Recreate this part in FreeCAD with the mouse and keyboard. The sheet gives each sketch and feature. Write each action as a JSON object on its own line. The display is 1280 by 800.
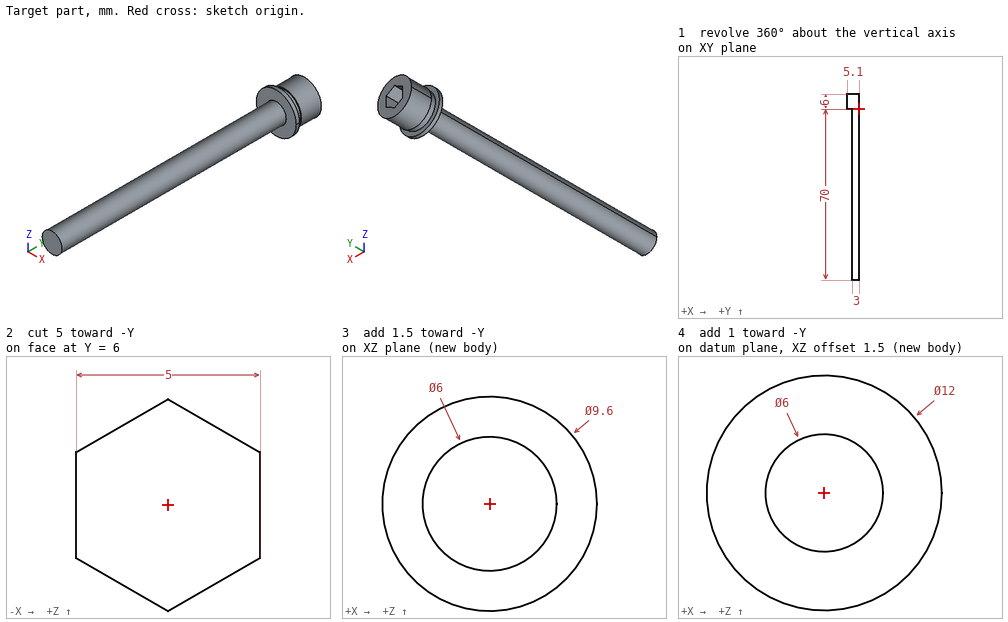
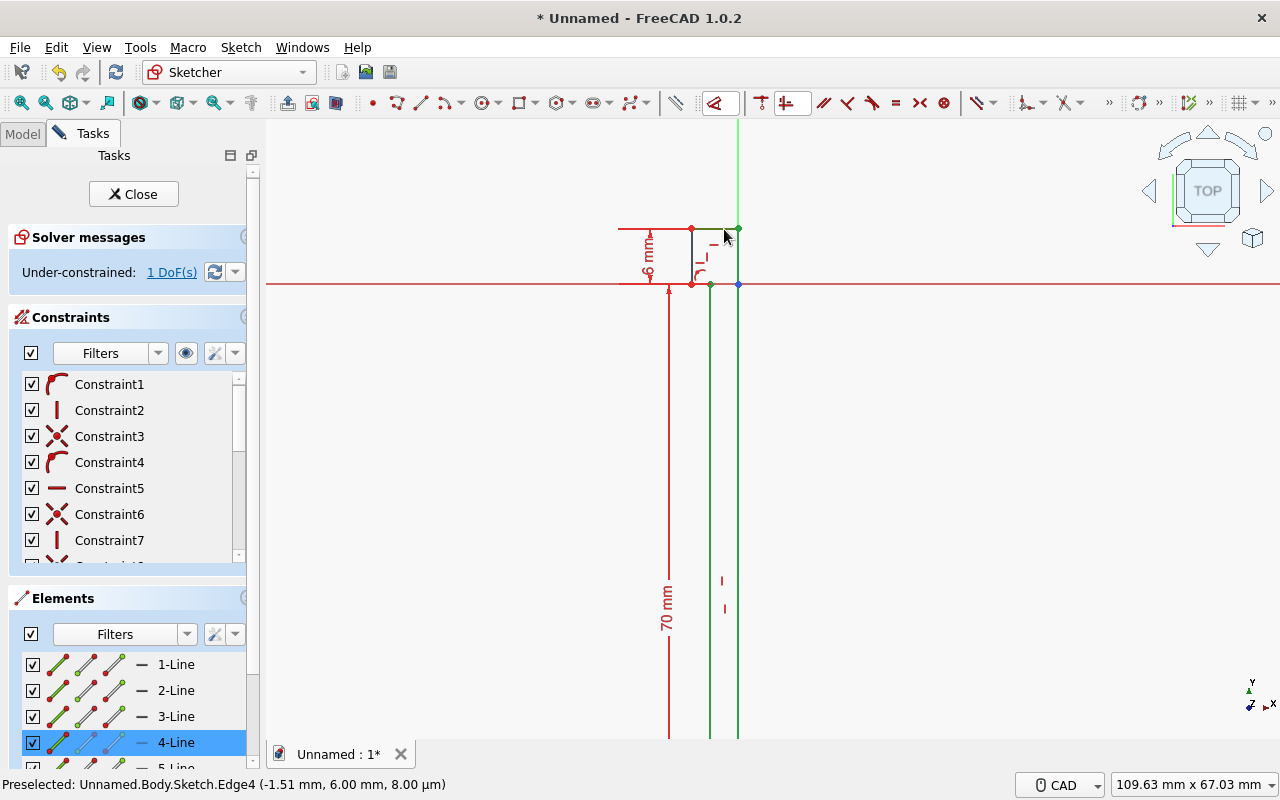
{"action": "key", "text": "l"}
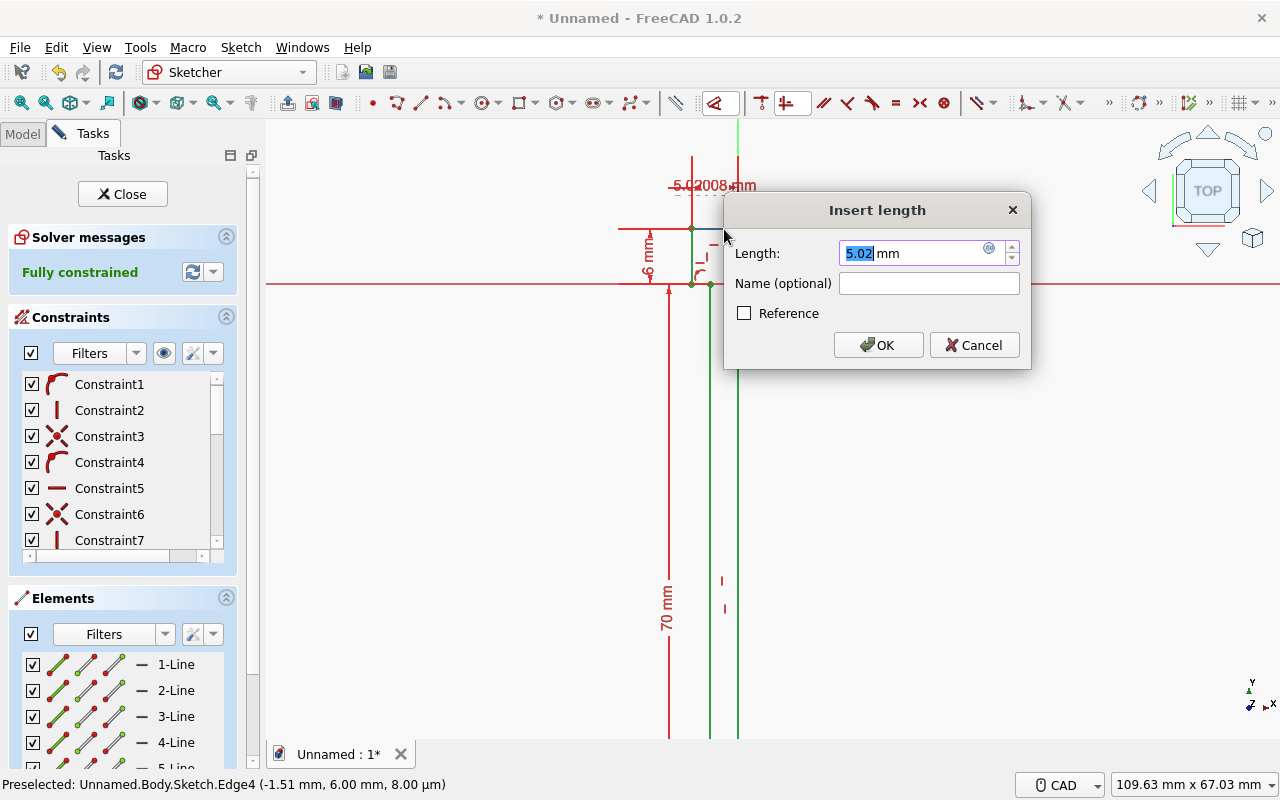
{"action": "type", "text": "5.1"}
{"action": "key", "text": "Return"}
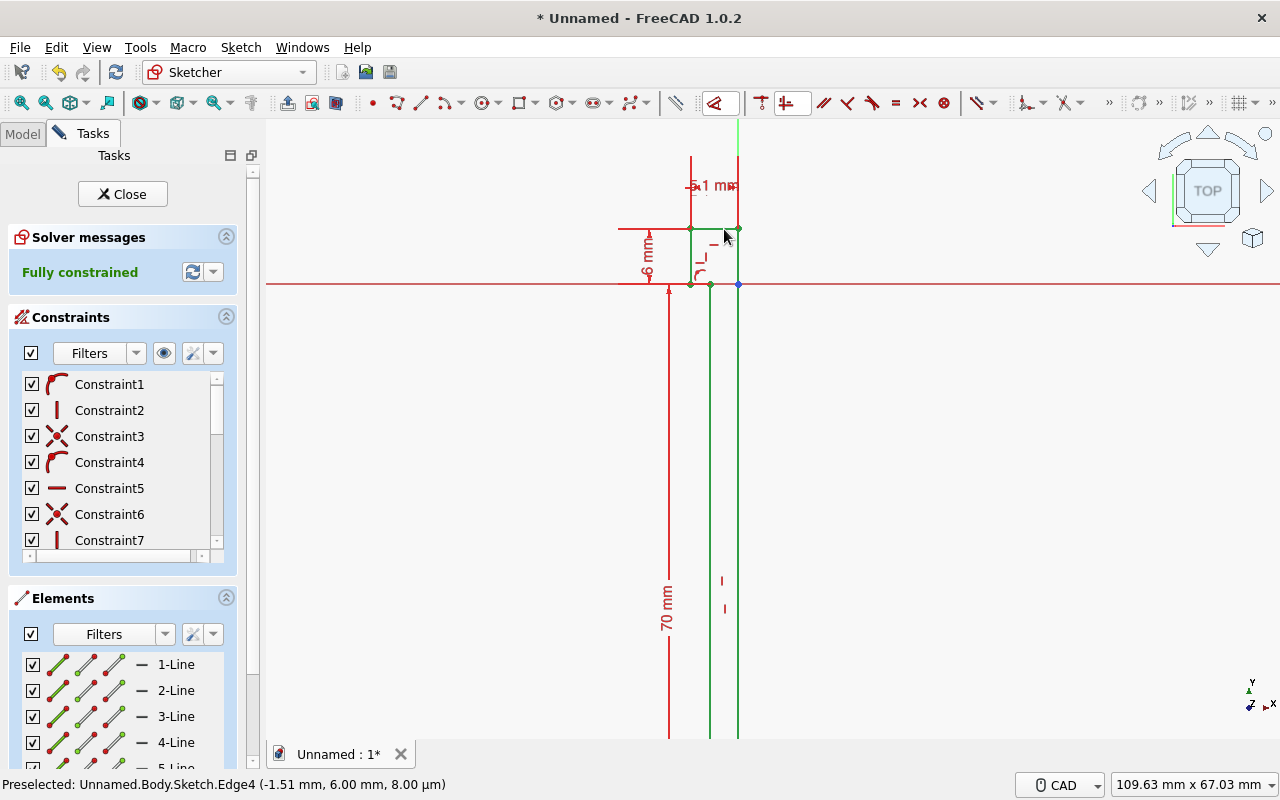
{"action": "left_click", "coordinate": [123, 194]}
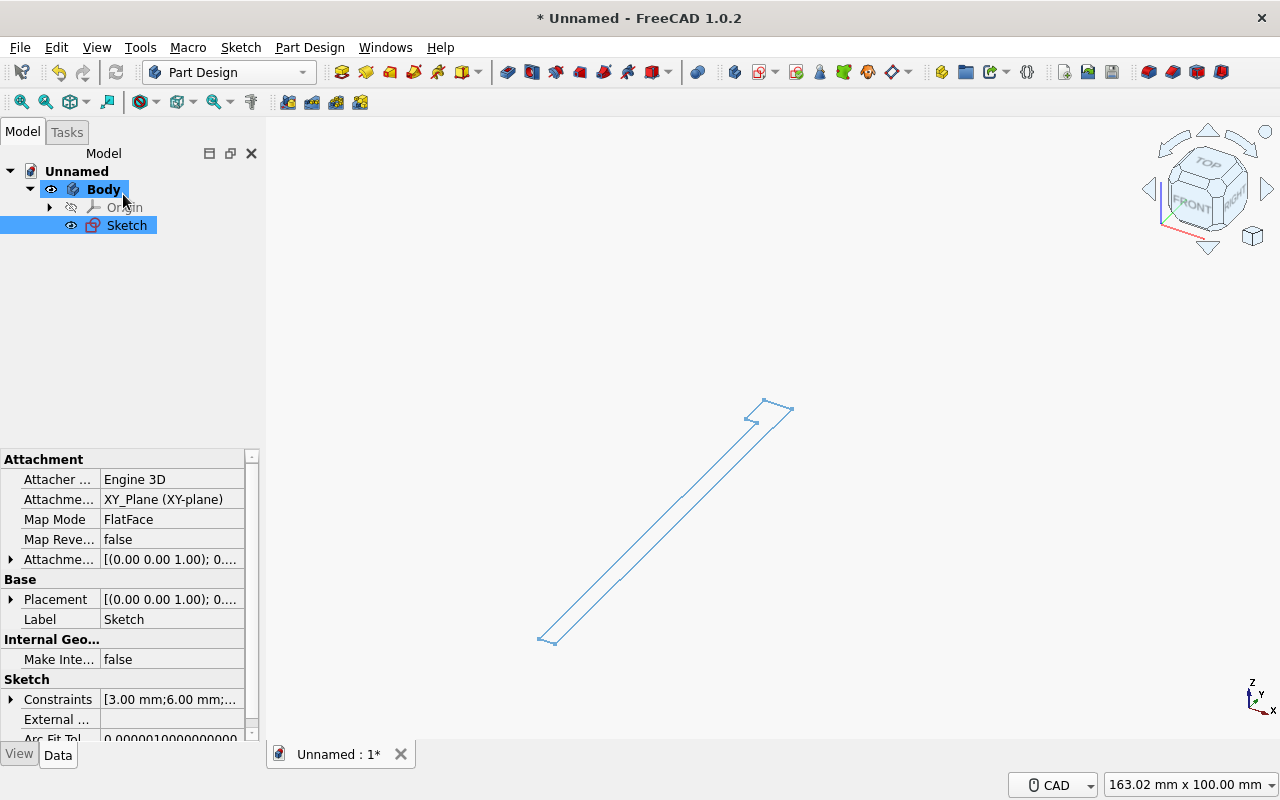
{"action": "left_click", "coordinate": [366, 72]}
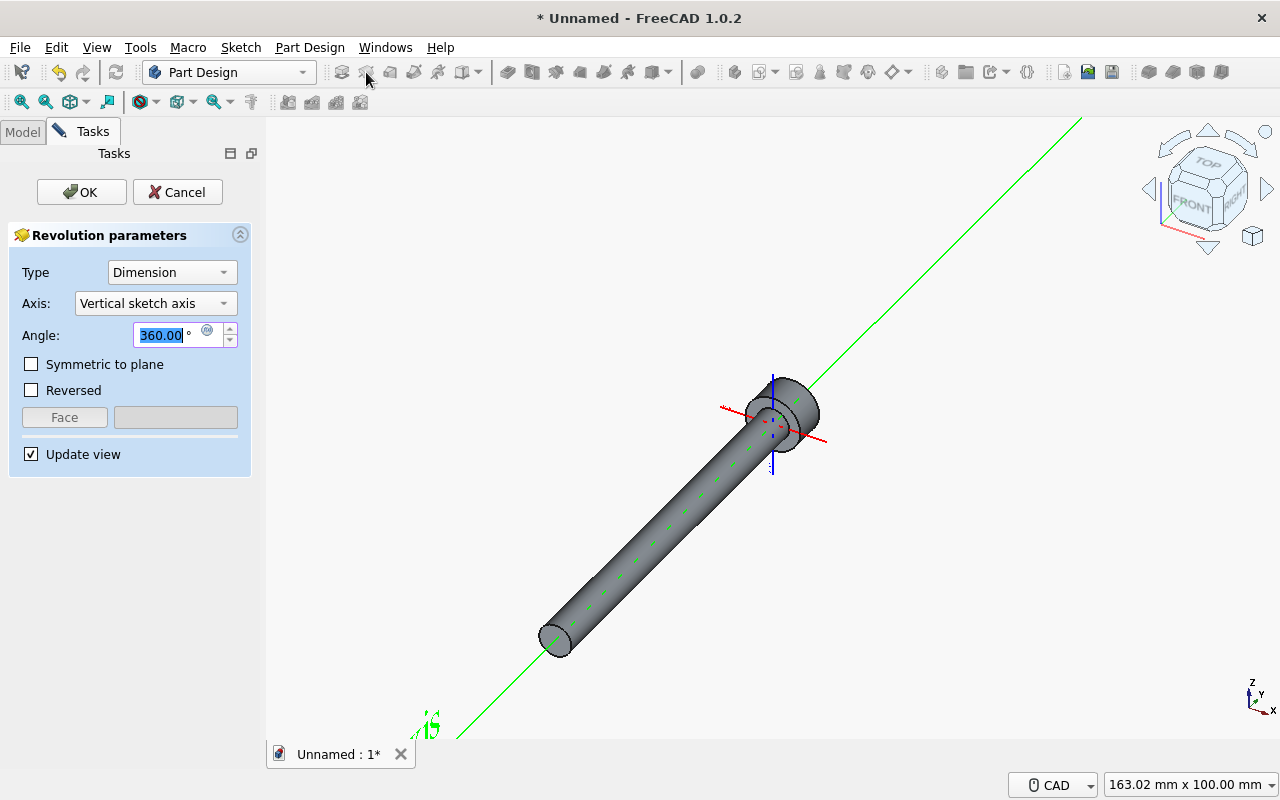
{"action": "left_click", "coordinate": [82, 192]}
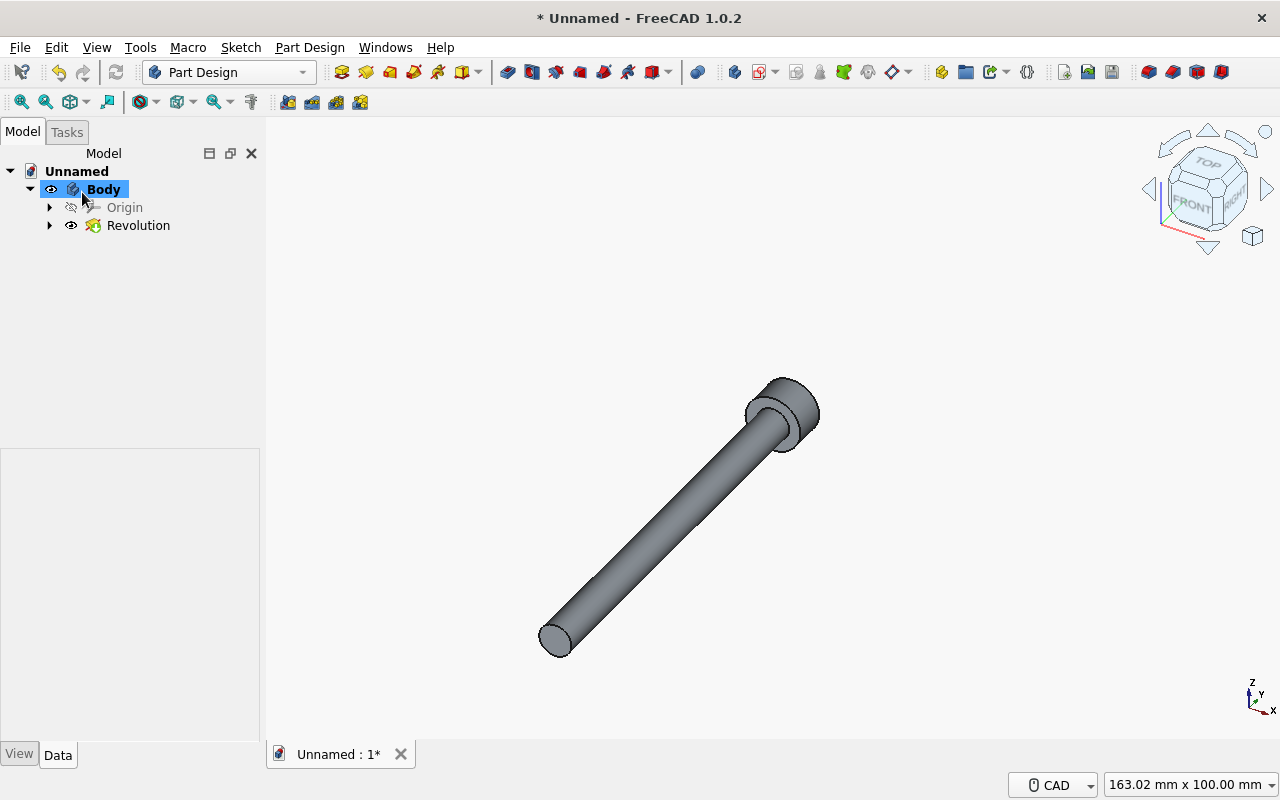
{"action": "key", "text": "4"}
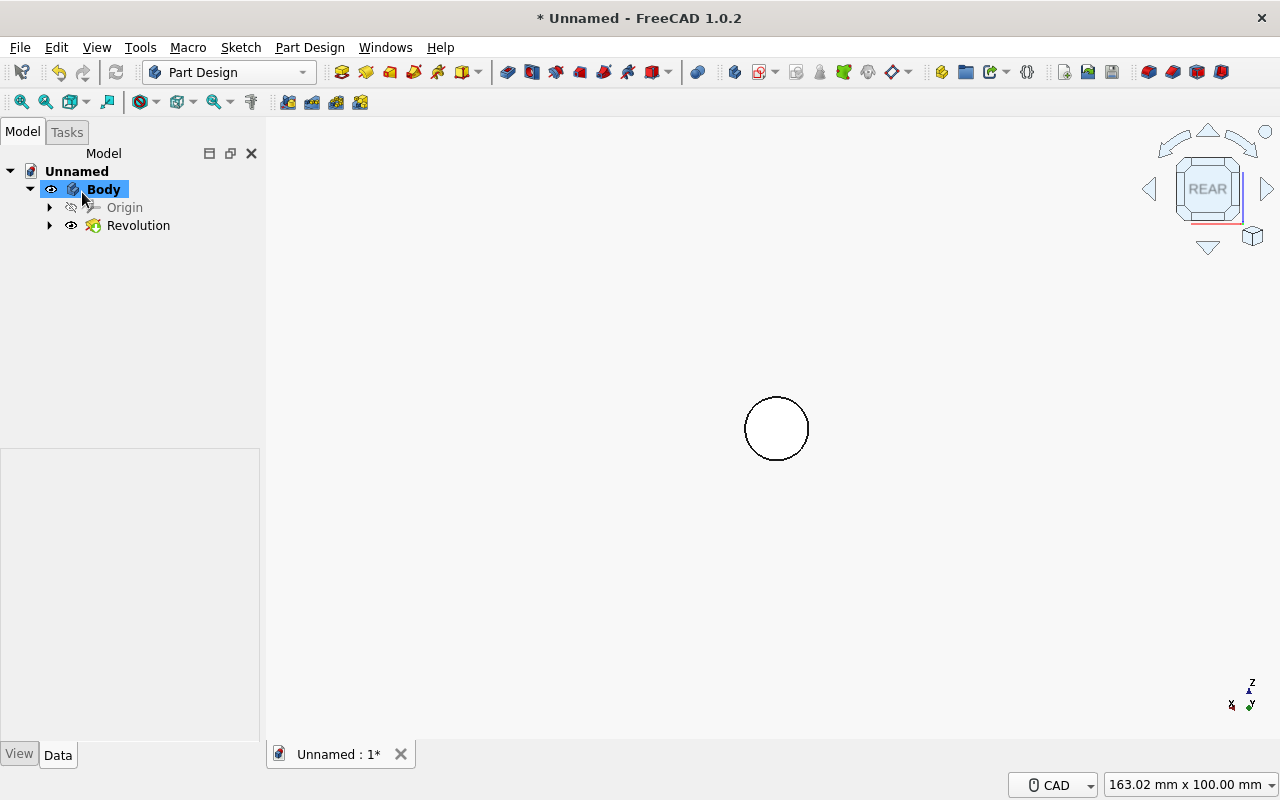
{"action": "key", "text": "v f"}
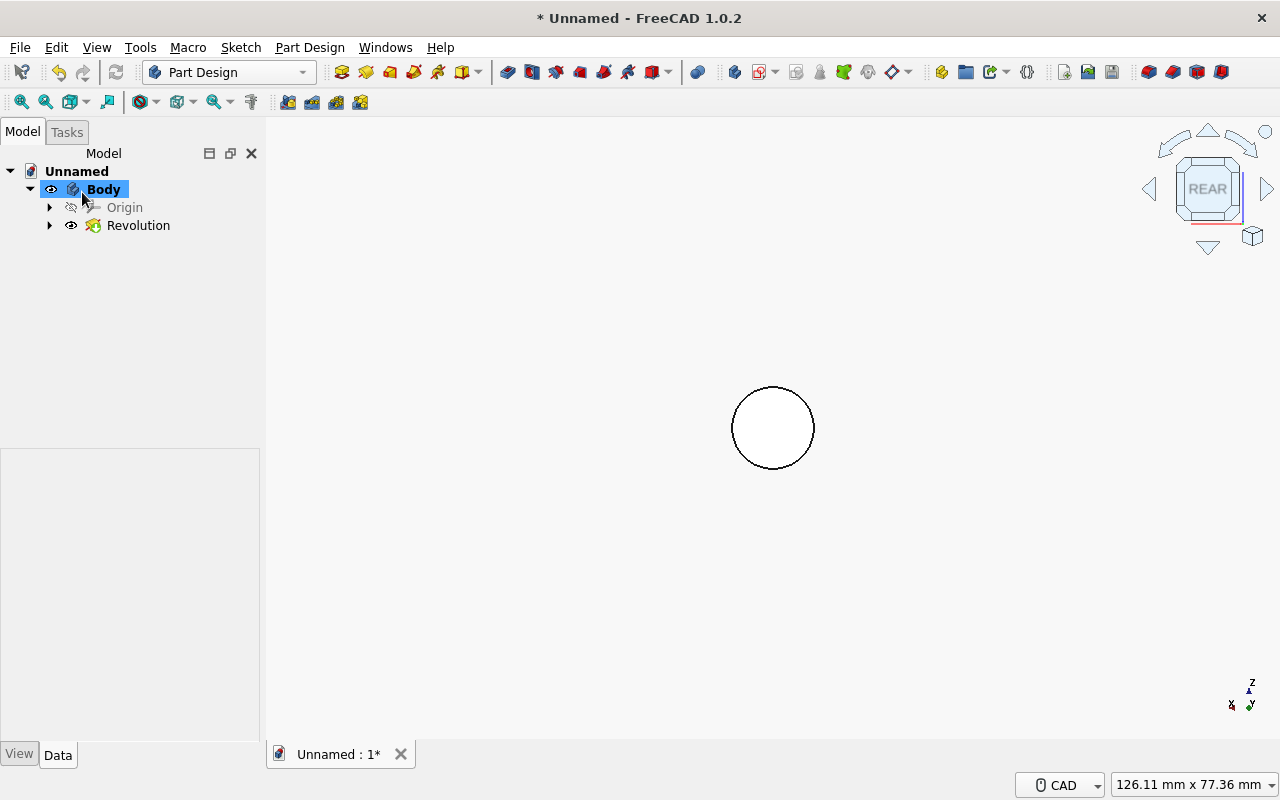
{"action": "left_click", "coordinate": [773, 427]}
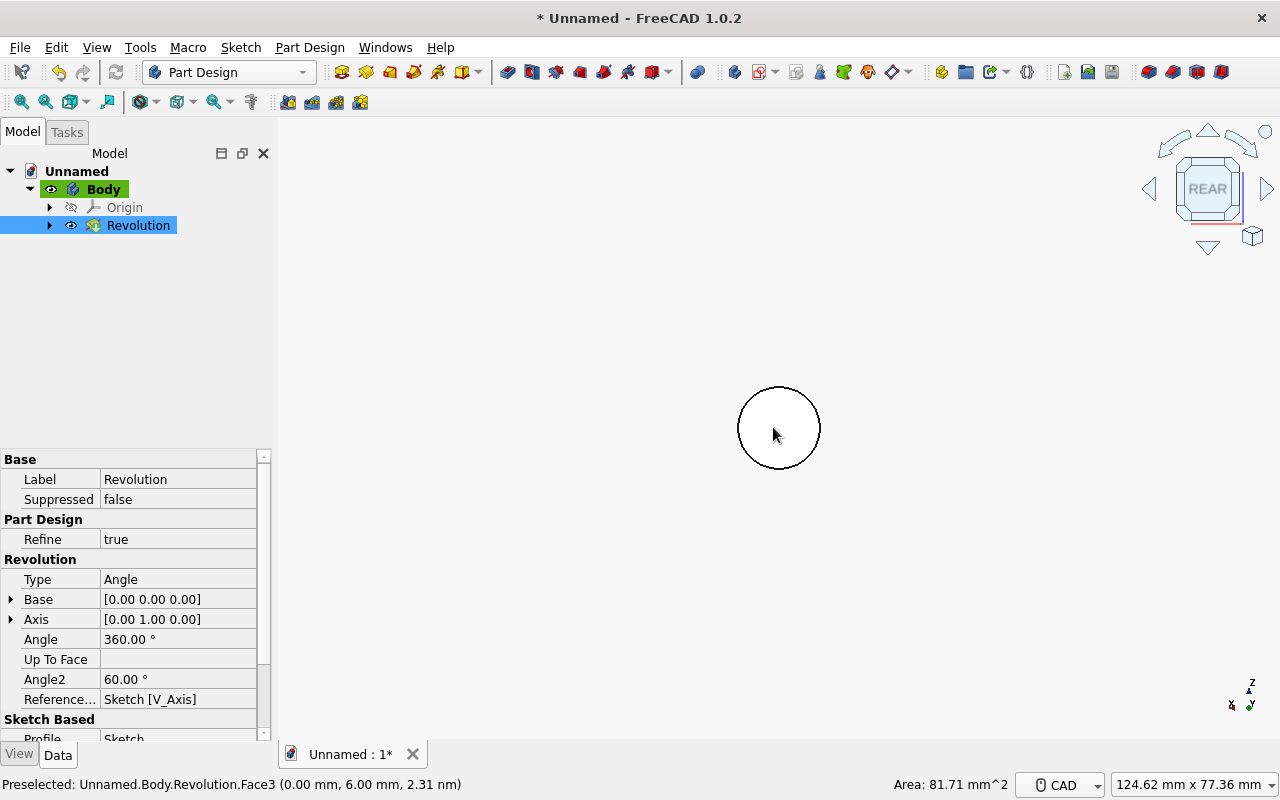
{"action": "left_click", "coordinate": [760, 72]}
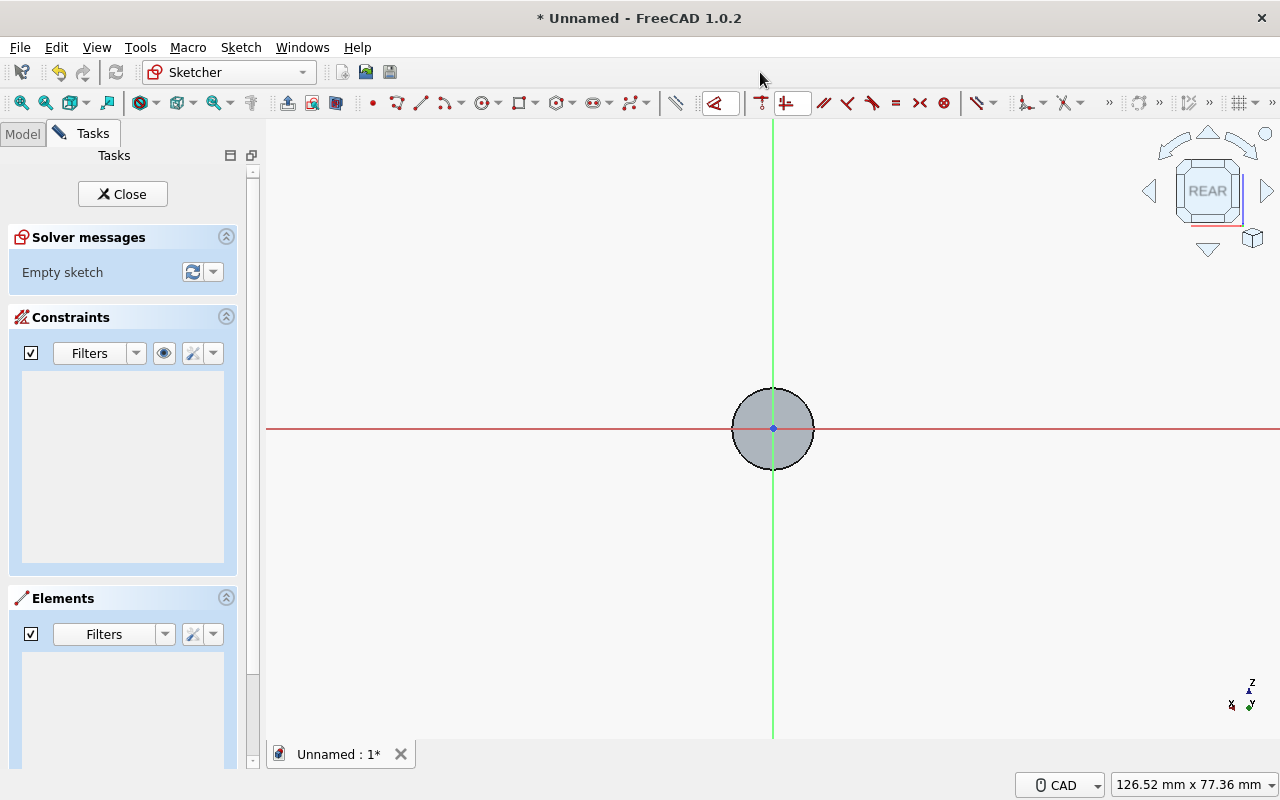
{"action": "scroll", "coordinate": [782, 429], "scroll_direction": "up", "scroll_amount": 11}